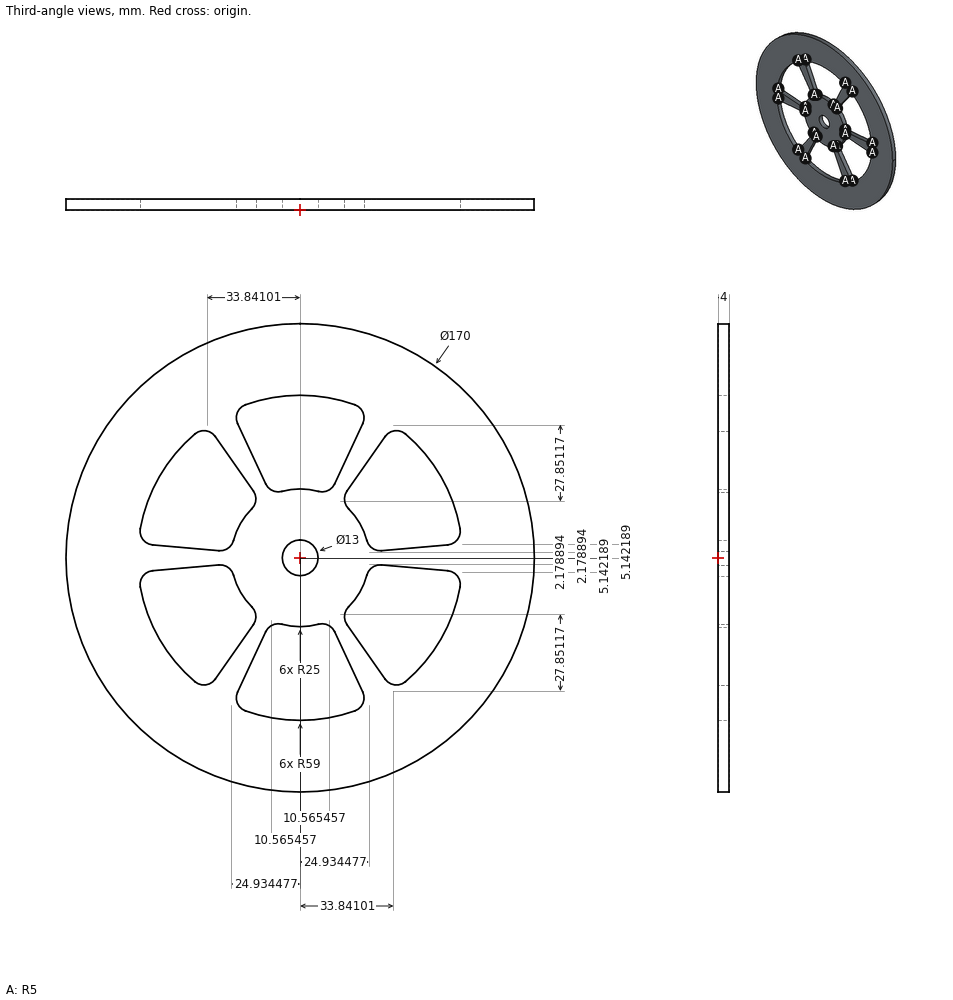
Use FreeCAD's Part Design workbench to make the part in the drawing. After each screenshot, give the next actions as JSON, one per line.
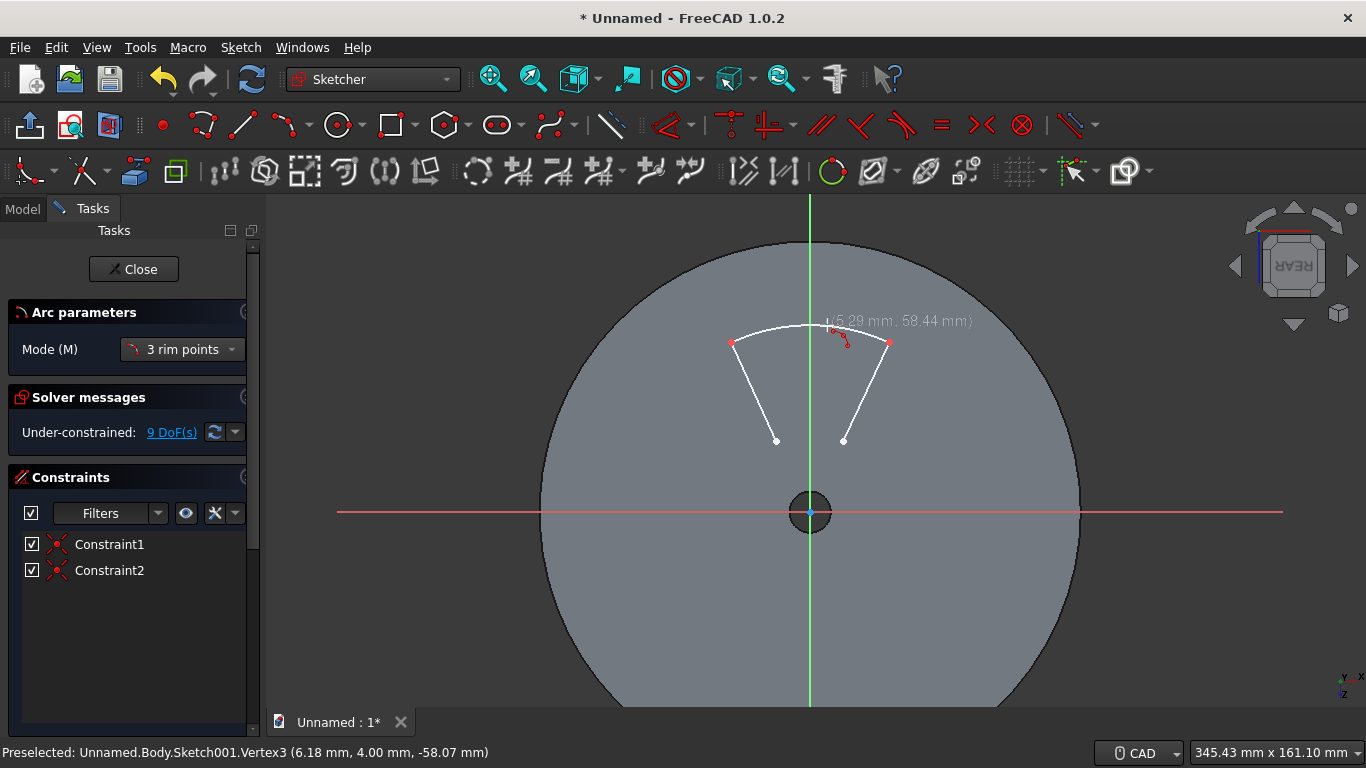
{"action": "left_click", "coordinate": [776, 441]}
{"action": "left_click", "coordinate": [843, 441]}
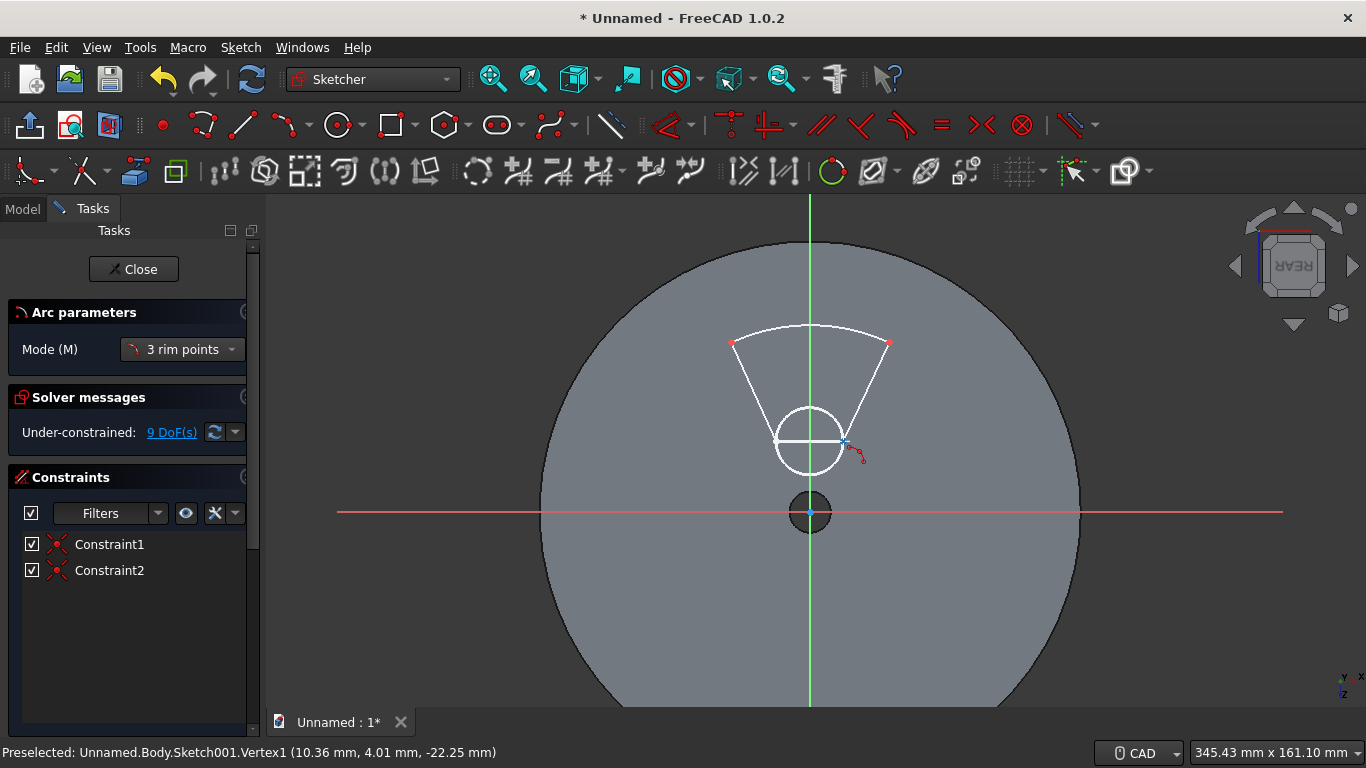
{"action": "scroll", "coordinate": [817, 433], "scroll_direction": "up", "scroll_amount": 5}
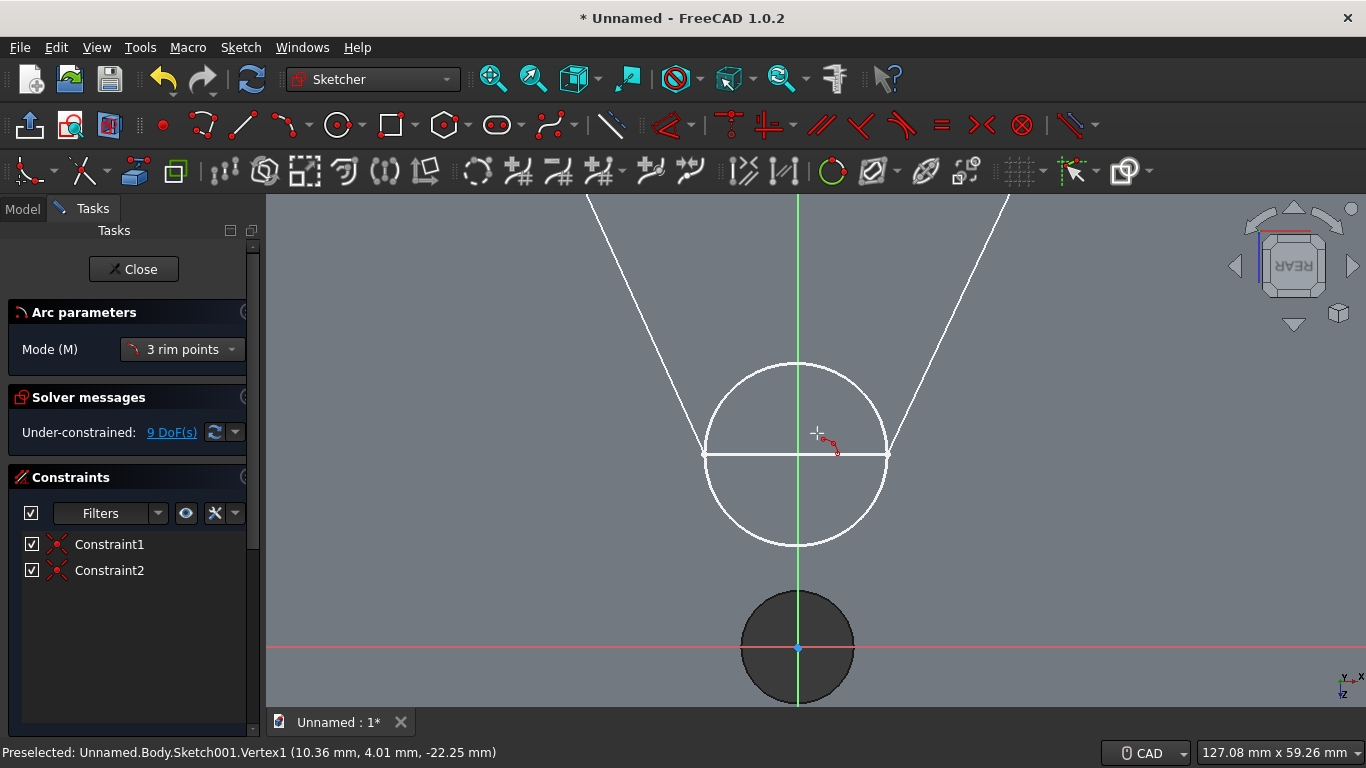
{"action": "left_click", "coordinate": [816, 432]}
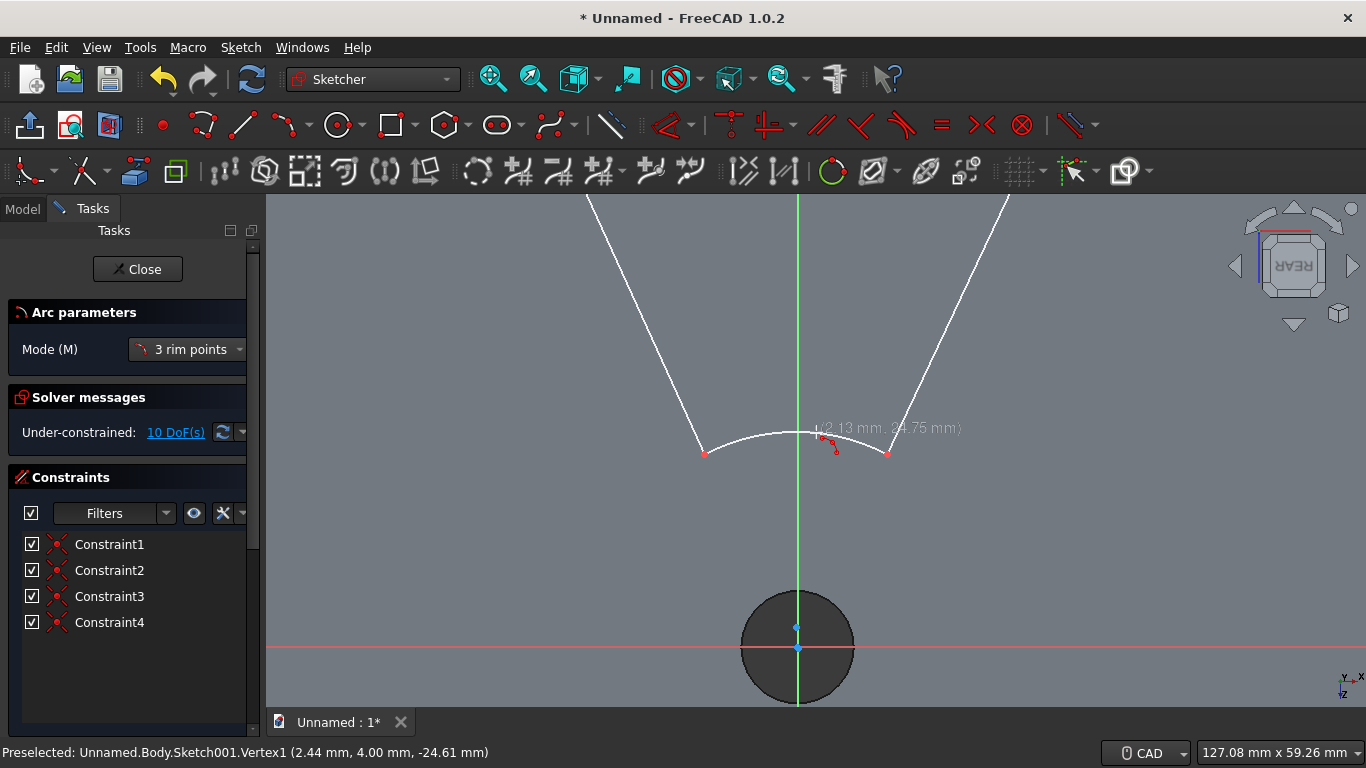
{"action": "left_click", "coordinate": [244, 126]}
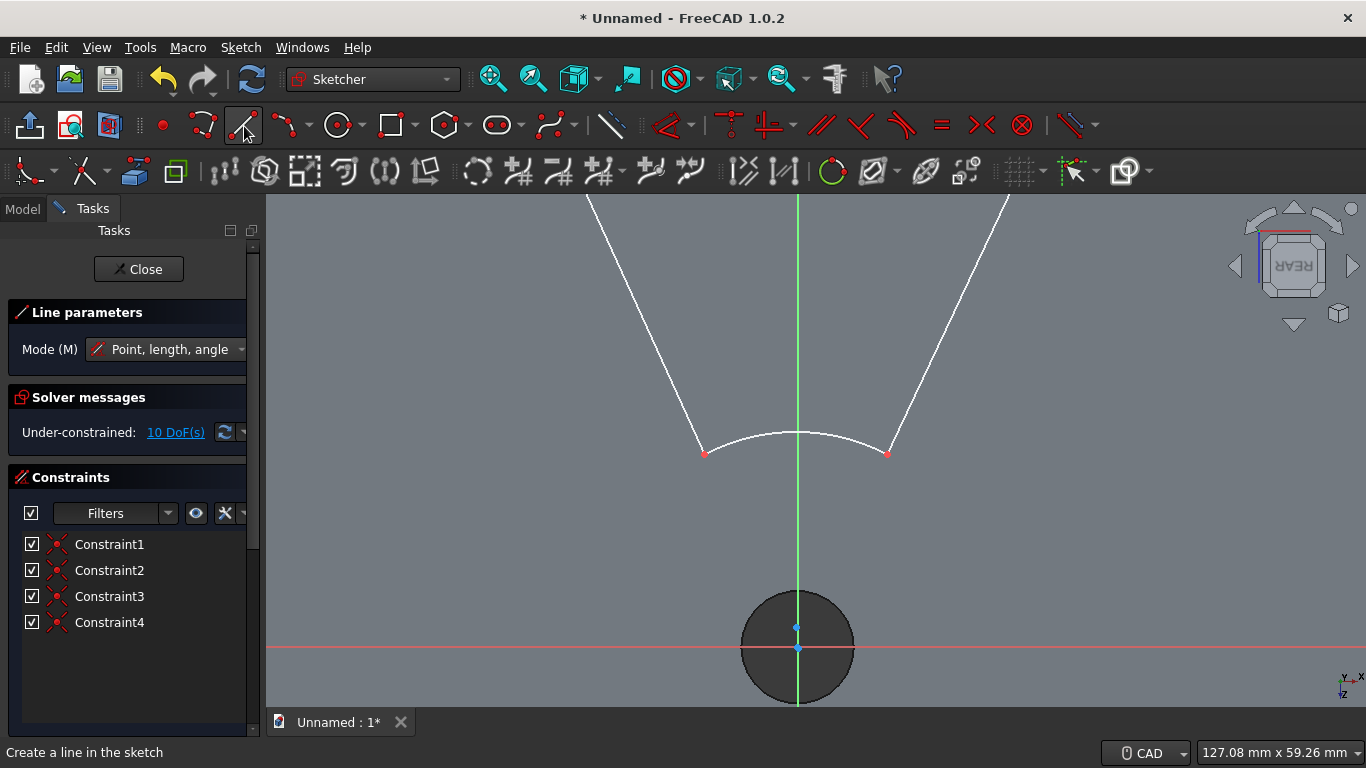
{"action": "scroll", "coordinate": [726, 366], "scroll_direction": "down", "scroll_amount": 6}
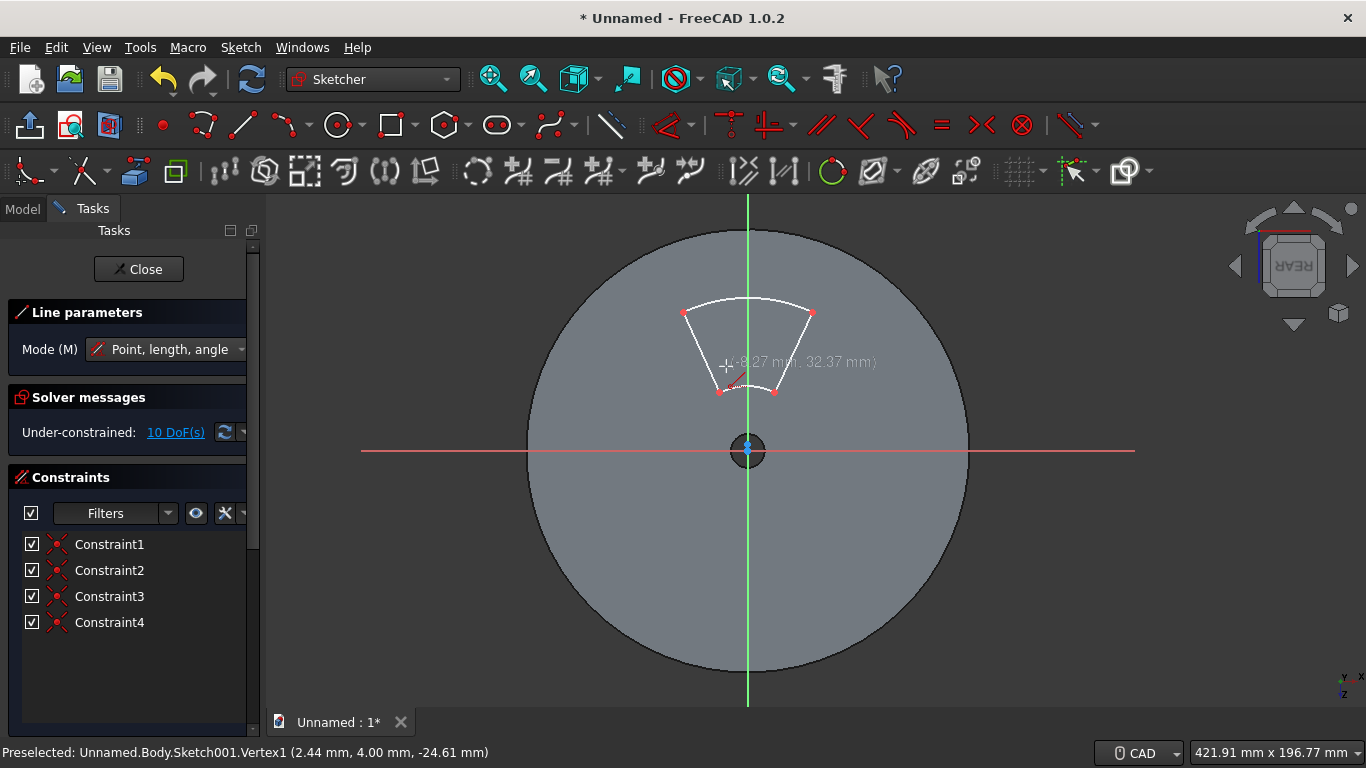
{"action": "left_click", "coordinate": [836, 325]}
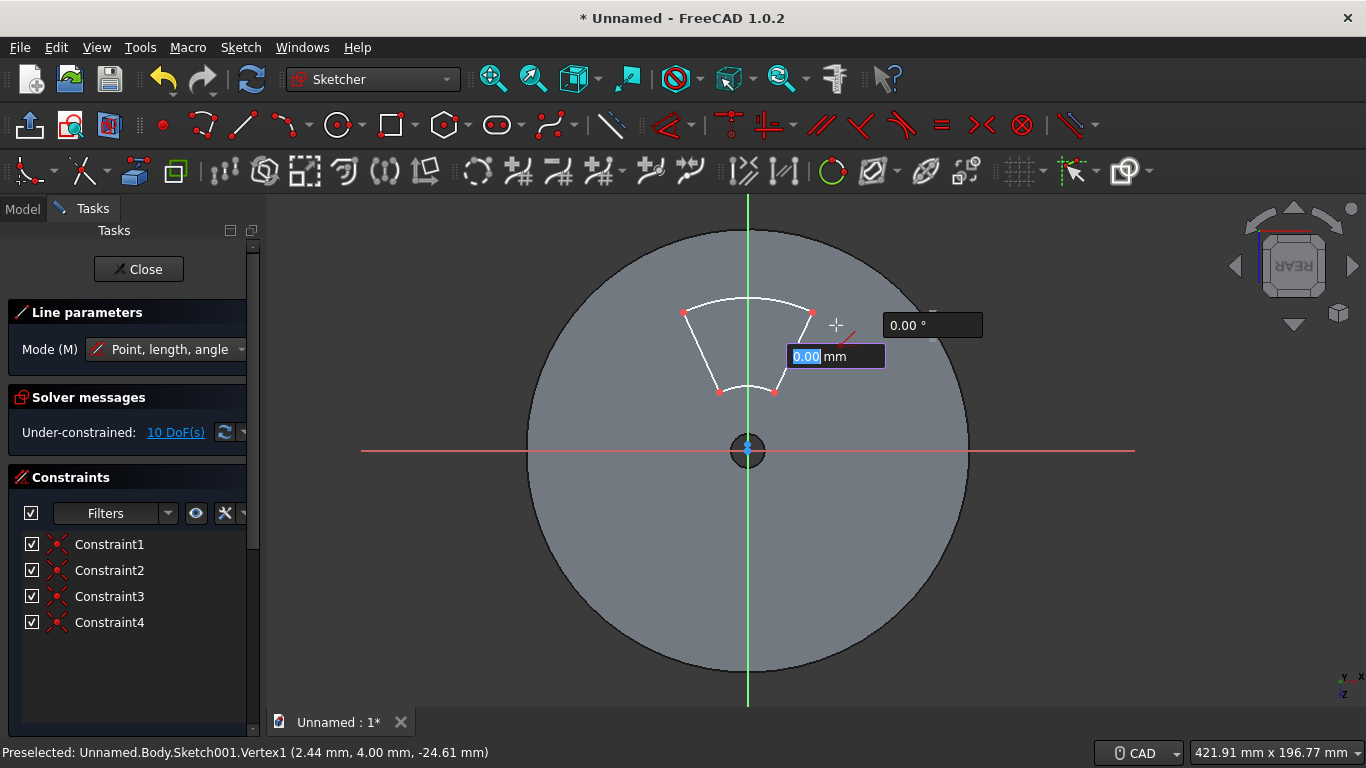
{"action": "scroll", "coordinate": [785, 398], "scroll_direction": "up", "scroll_amount": 2}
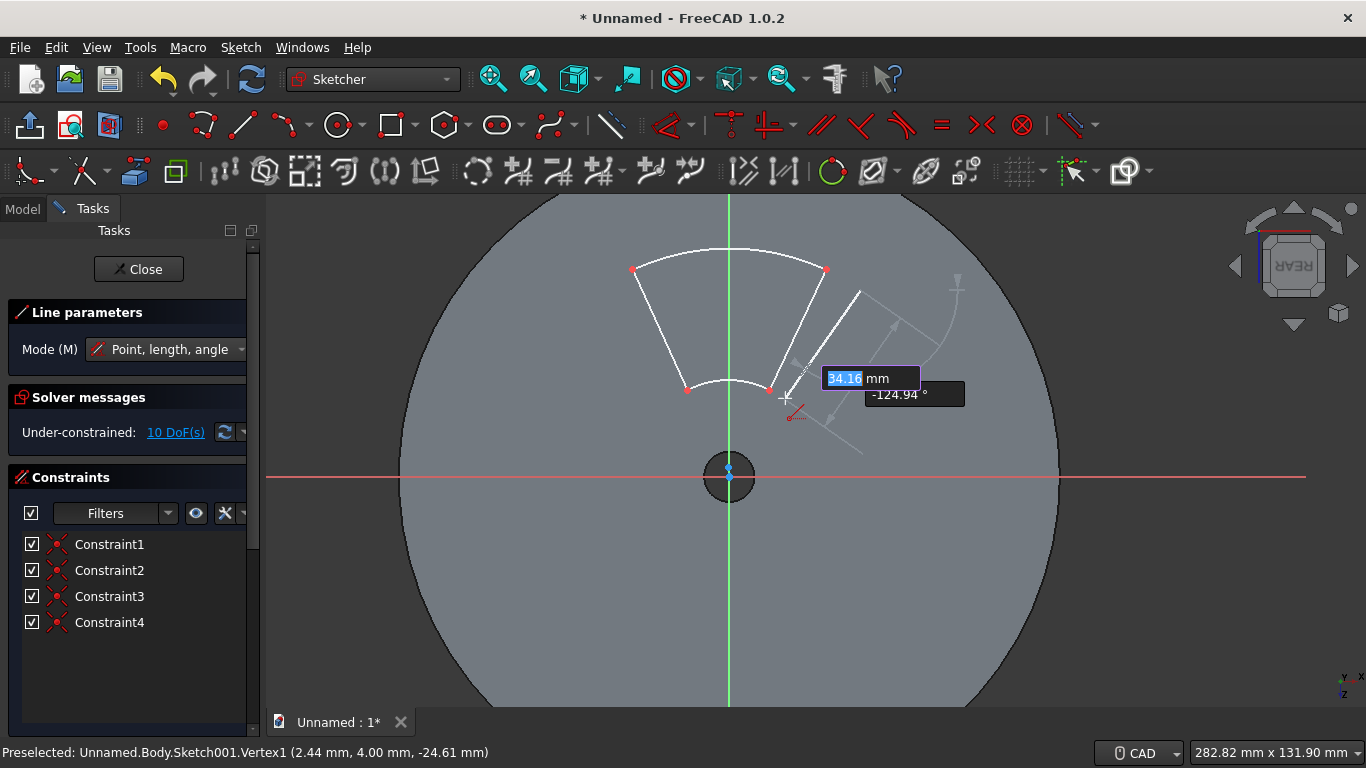
{"action": "left_click", "coordinate": [785, 397]}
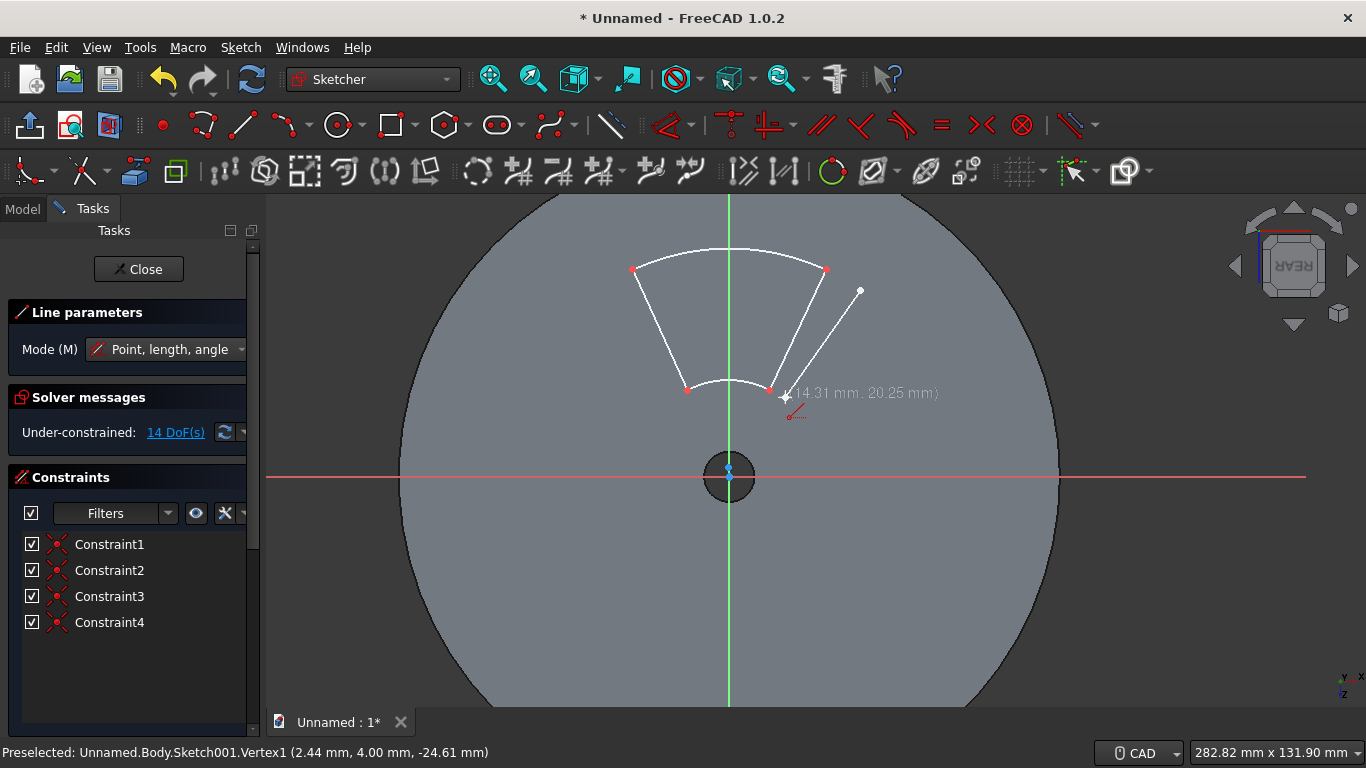
{"action": "scroll", "coordinate": [826, 468], "scroll_direction": "up", "scroll_amount": 4}